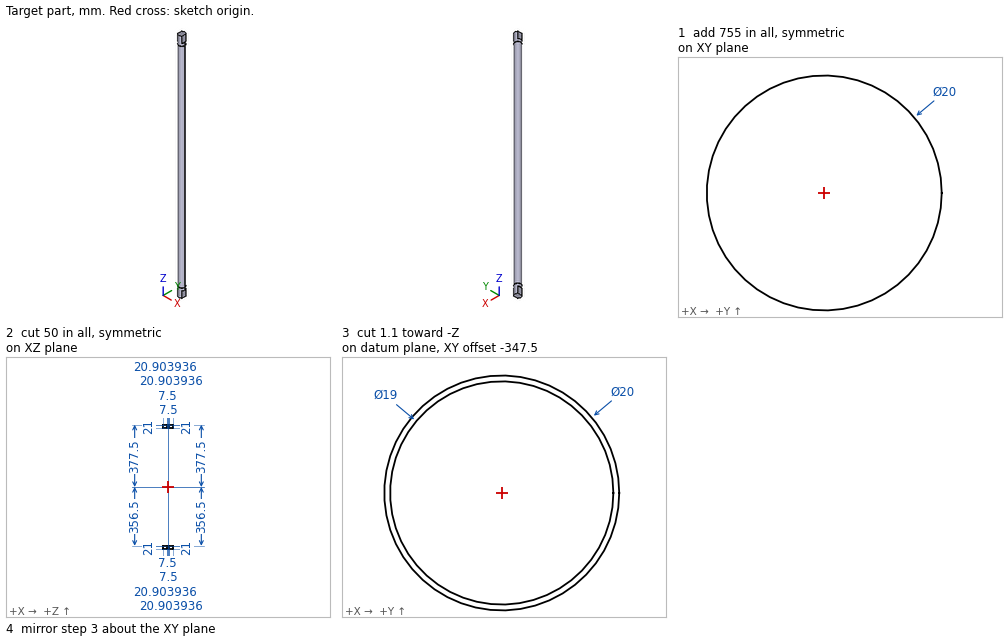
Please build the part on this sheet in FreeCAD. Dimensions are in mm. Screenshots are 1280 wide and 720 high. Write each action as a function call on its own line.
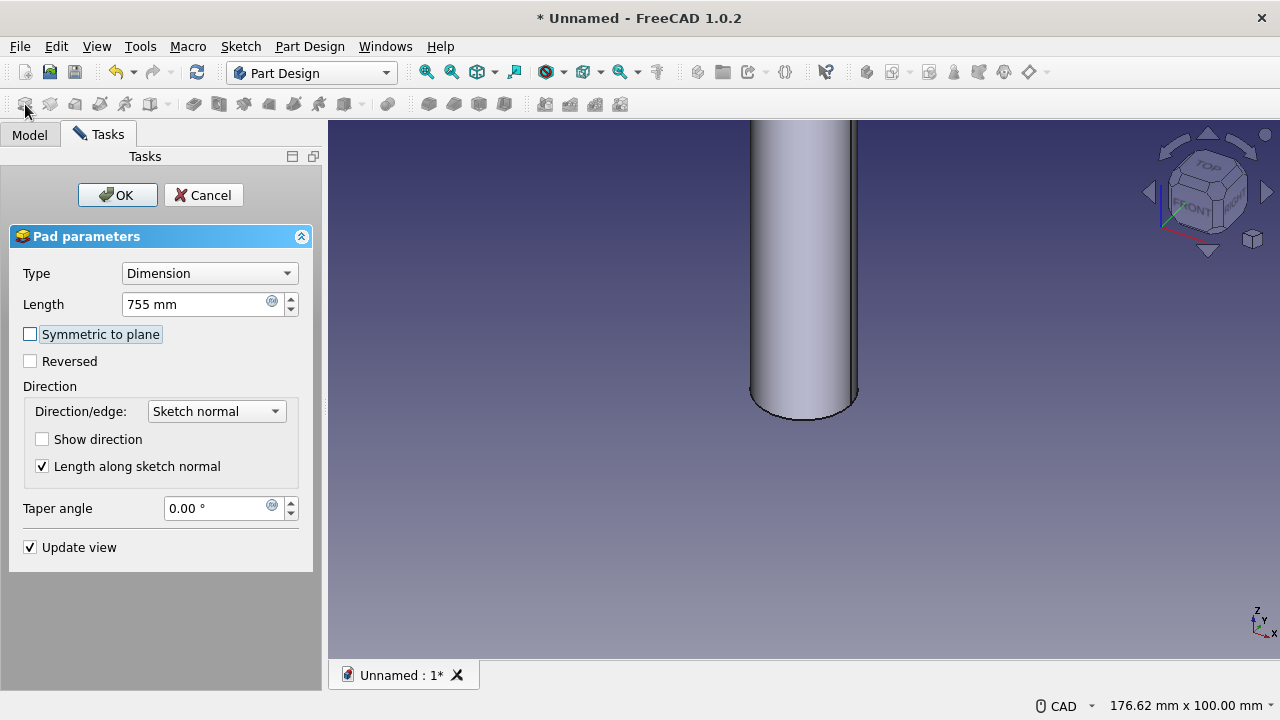
click(31, 334)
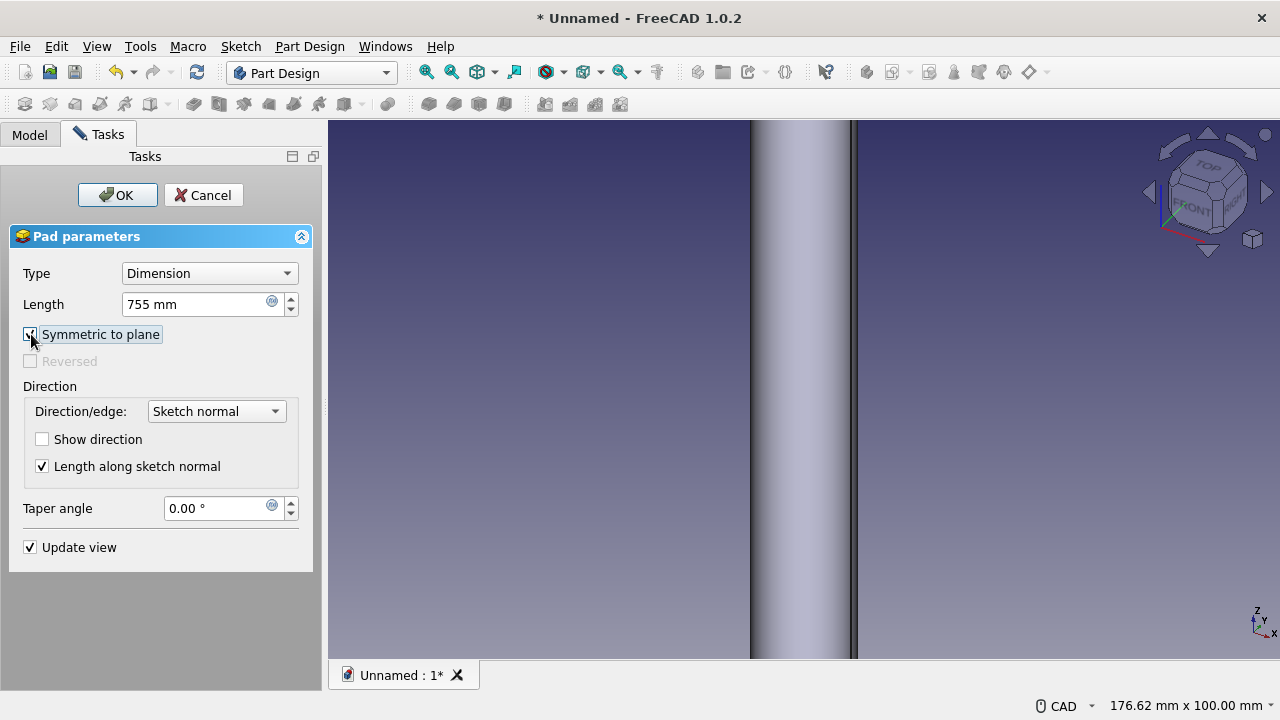
click(118, 195)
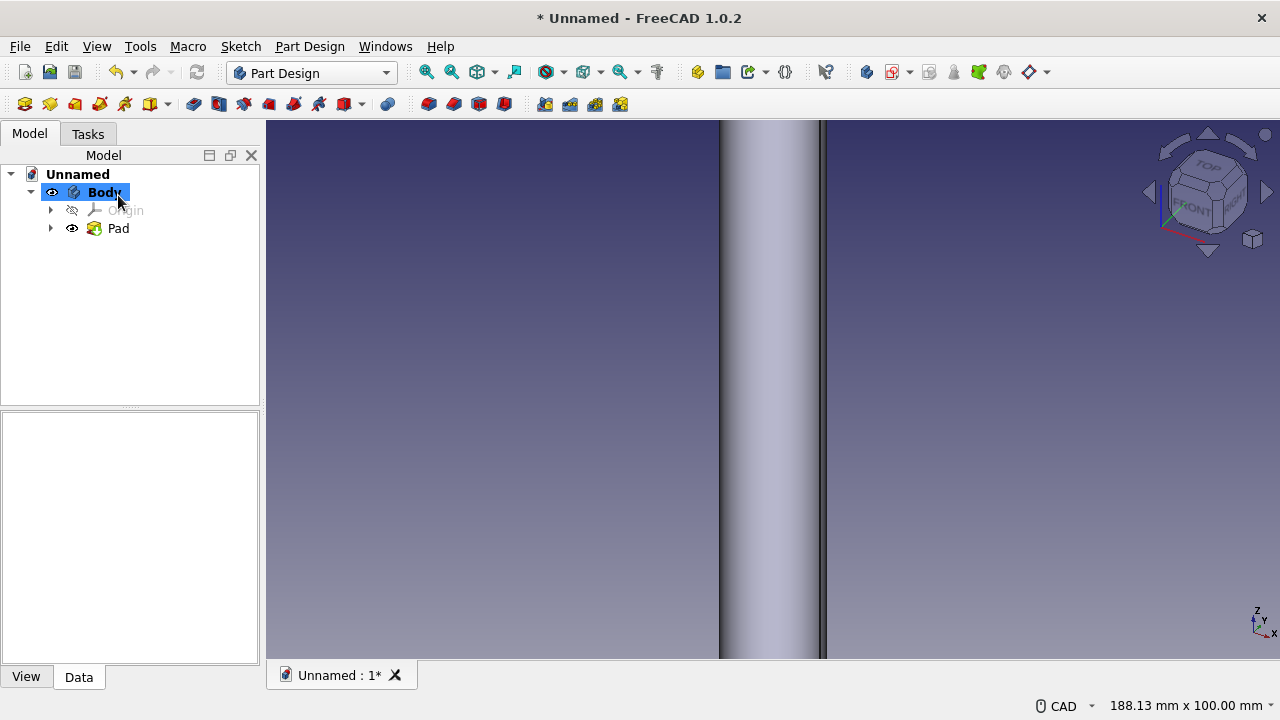
key(v)
key(f)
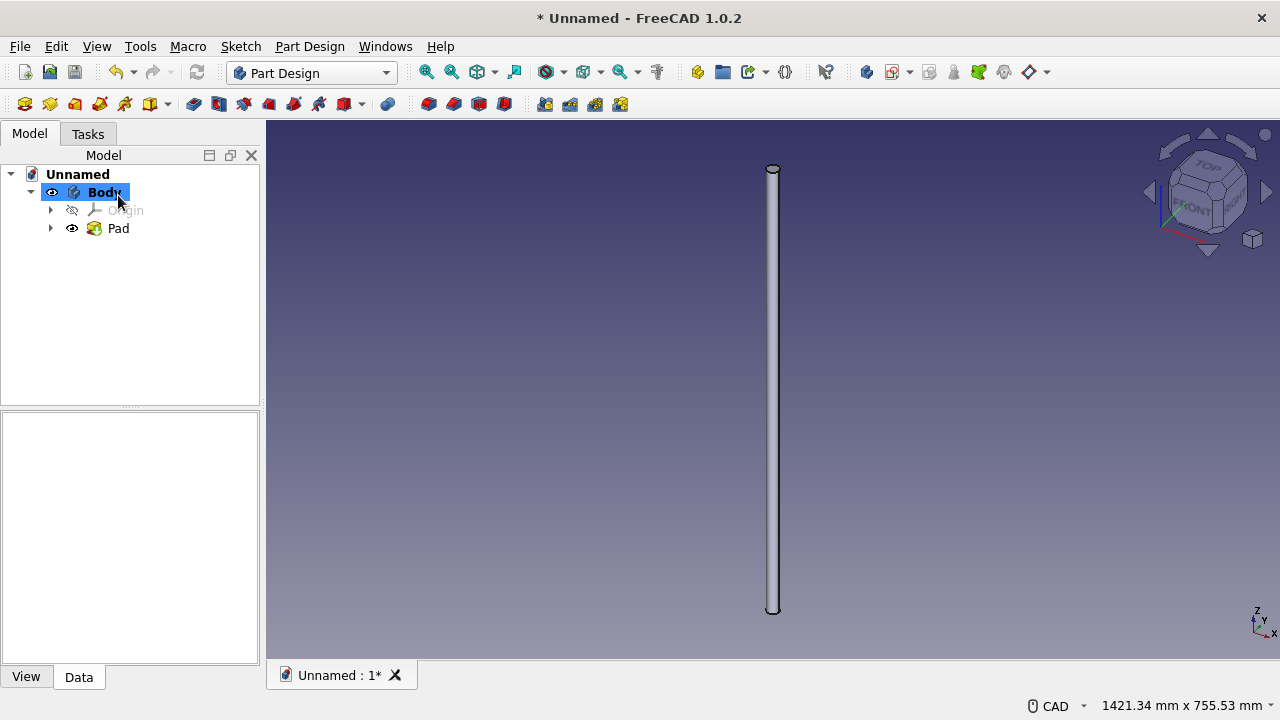
click(892, 72)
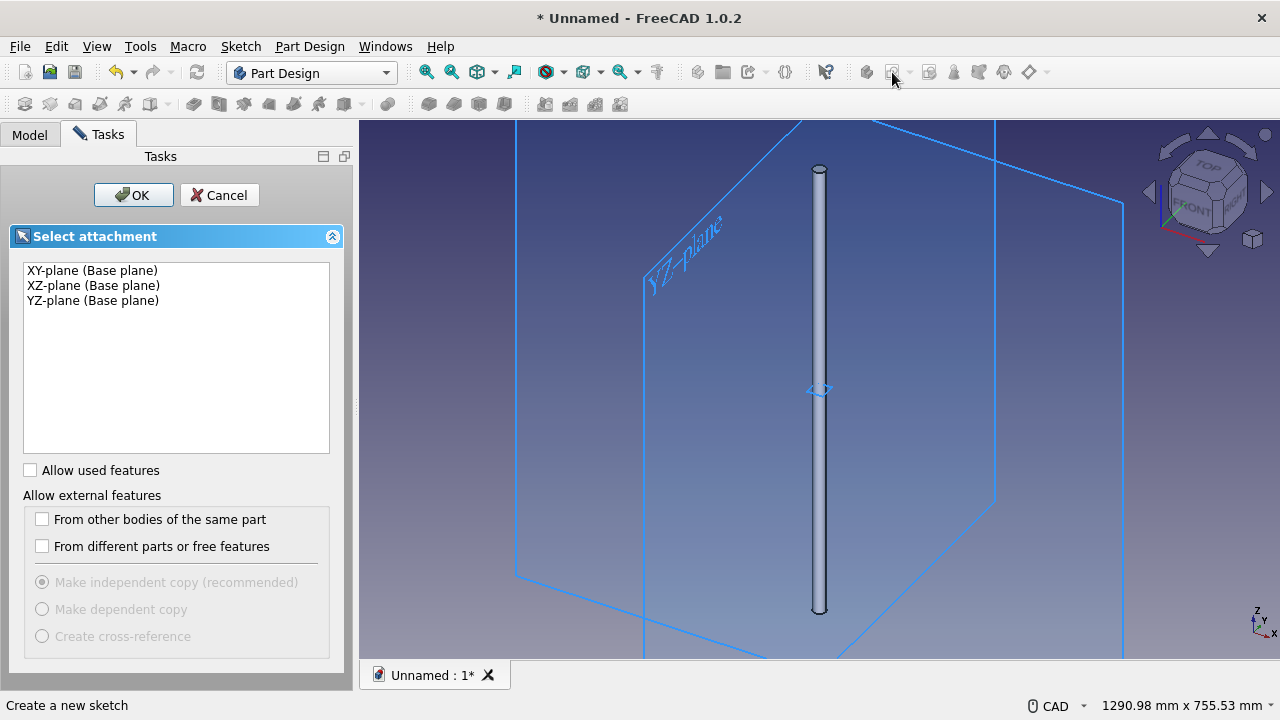
click(84, 286)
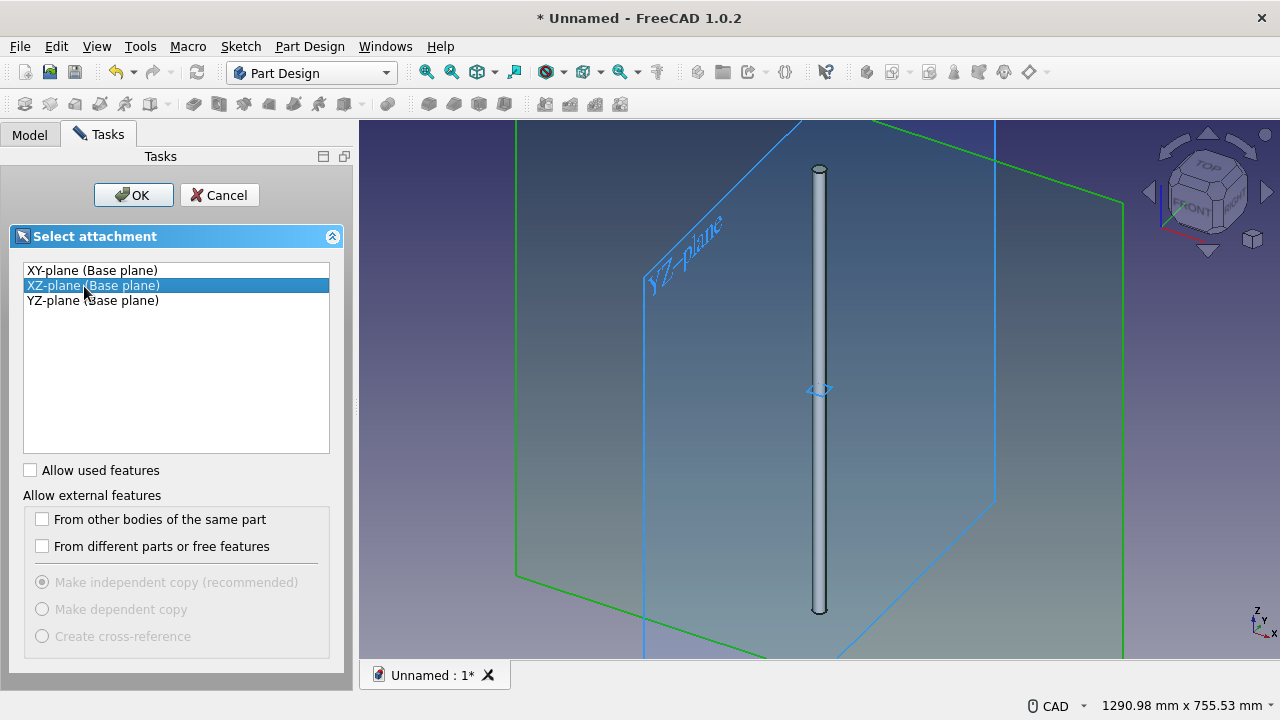
click(134, 195)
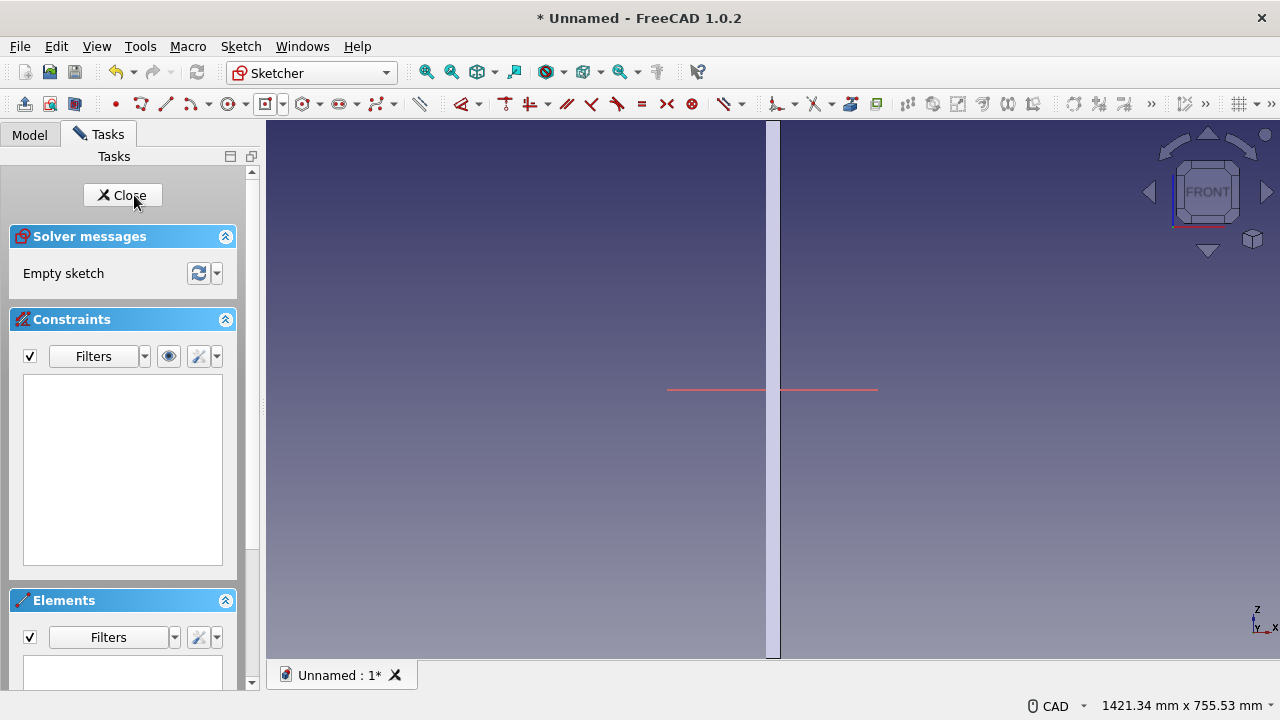
key(q)
key(s)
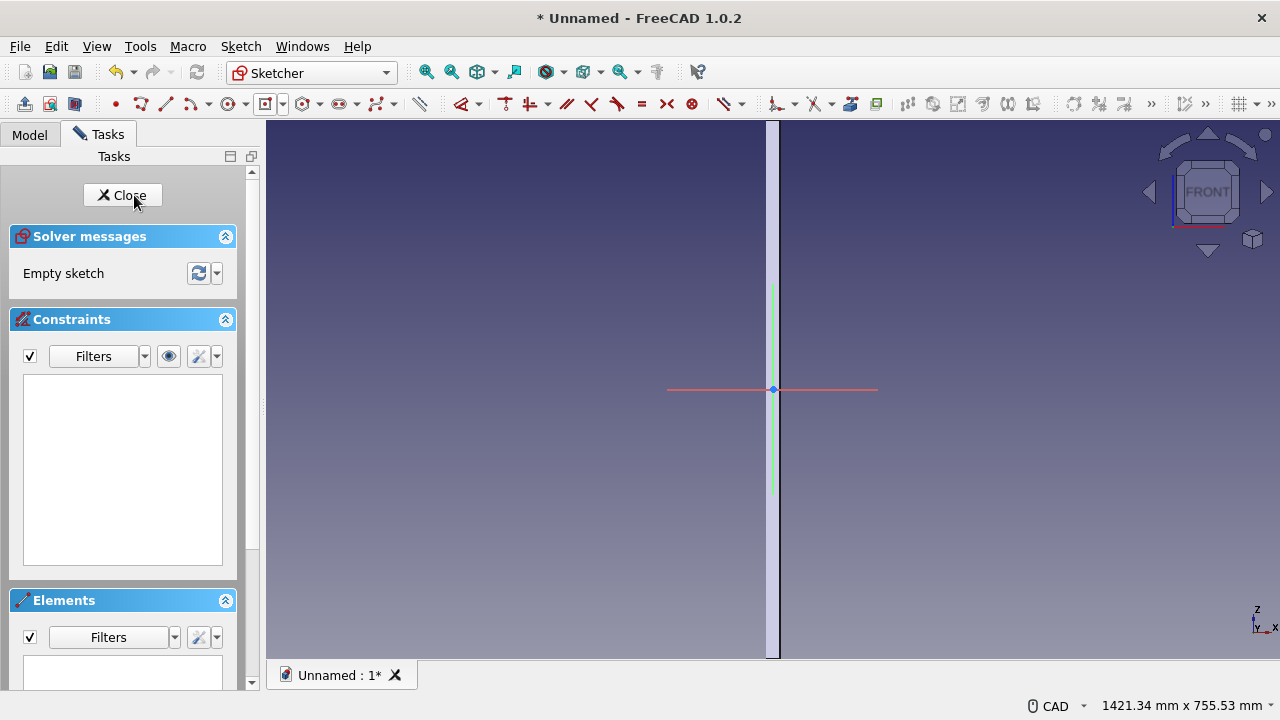
scroll(565, 389, down, 2)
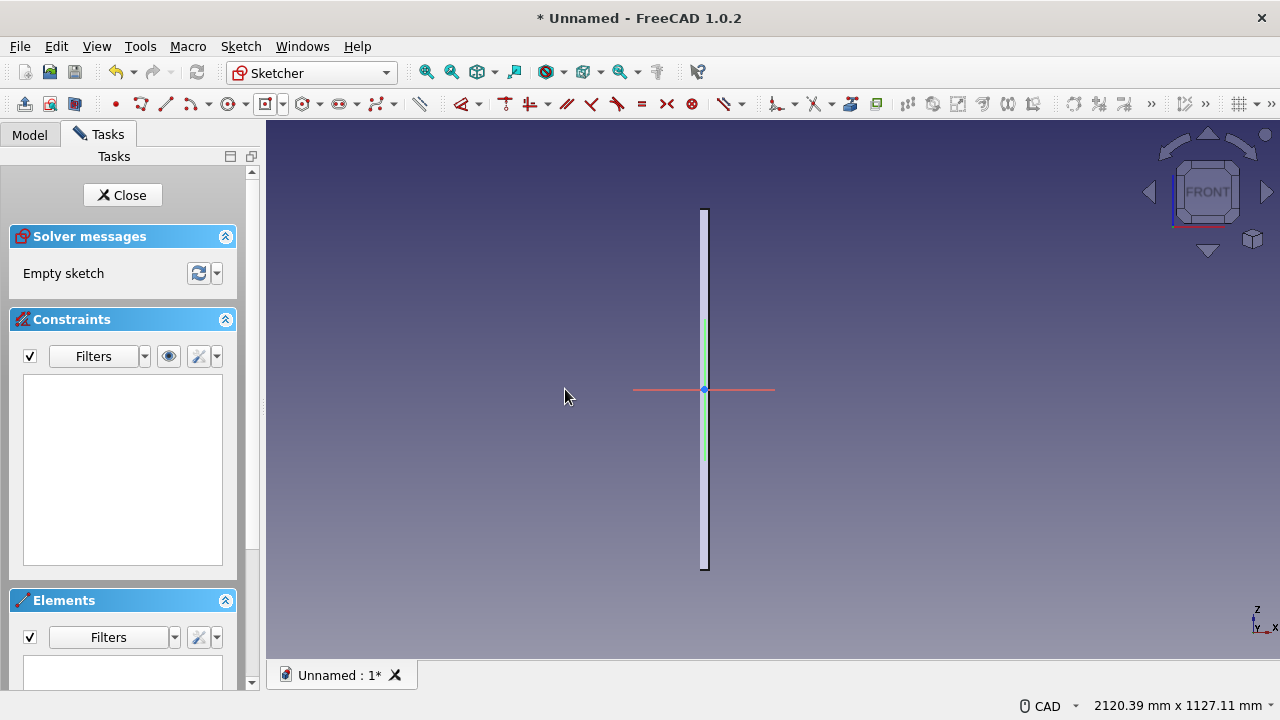
key(g)
key(r)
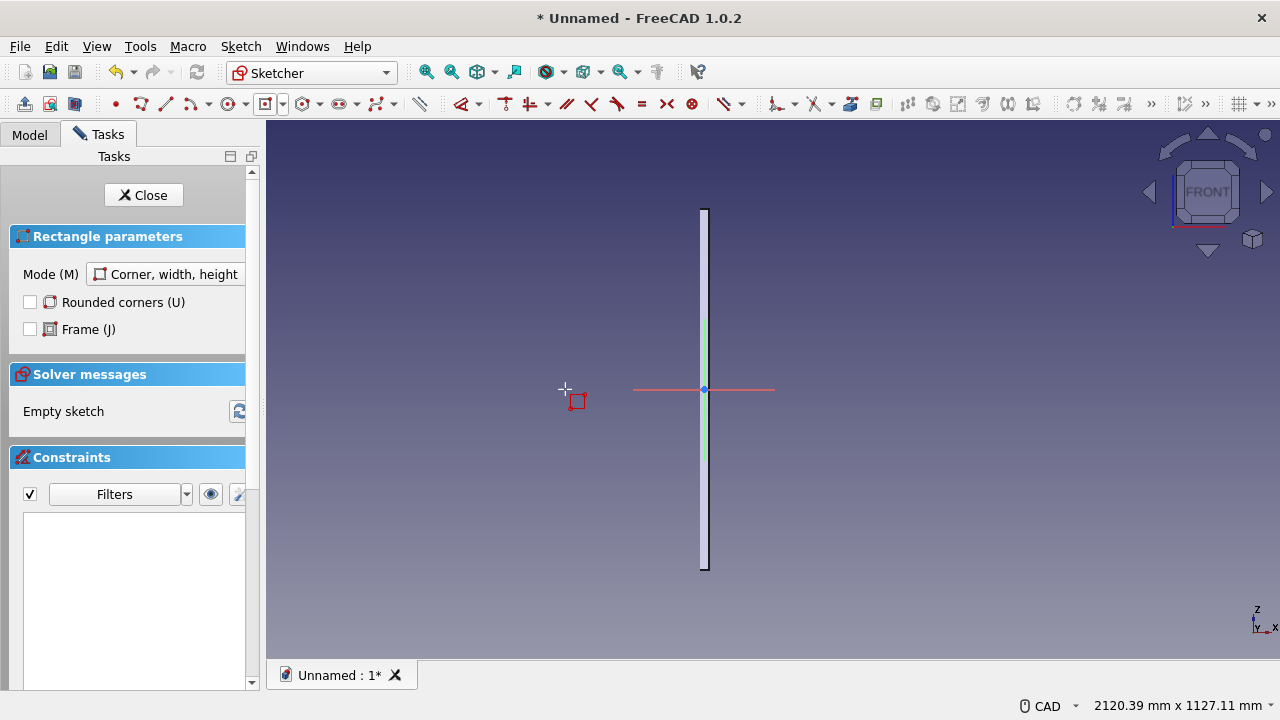
scroll(691, 560, up, 3)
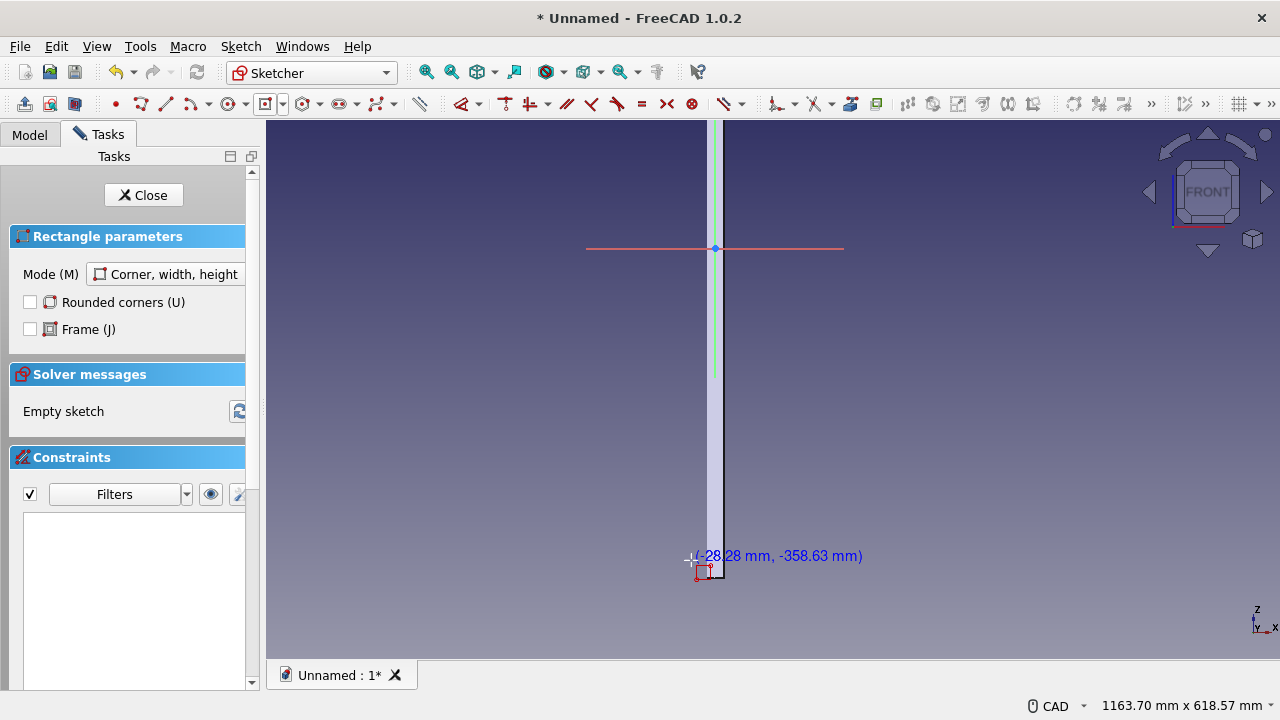
click(691, 559)